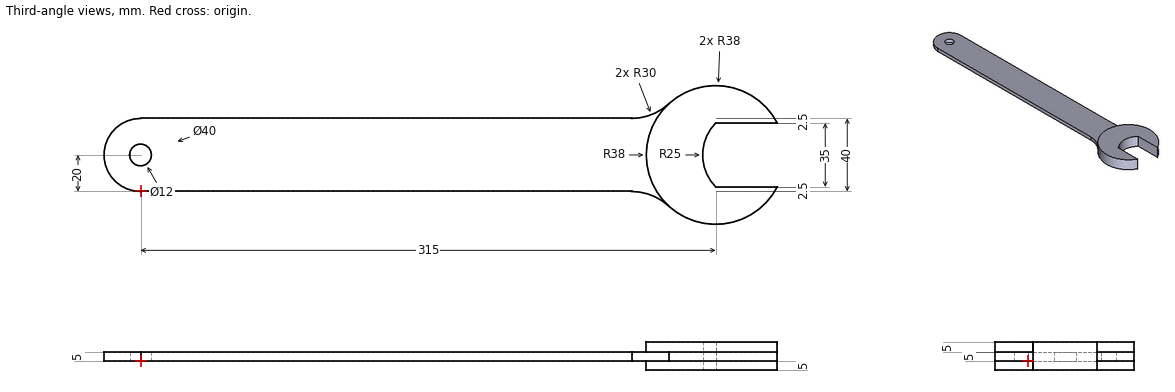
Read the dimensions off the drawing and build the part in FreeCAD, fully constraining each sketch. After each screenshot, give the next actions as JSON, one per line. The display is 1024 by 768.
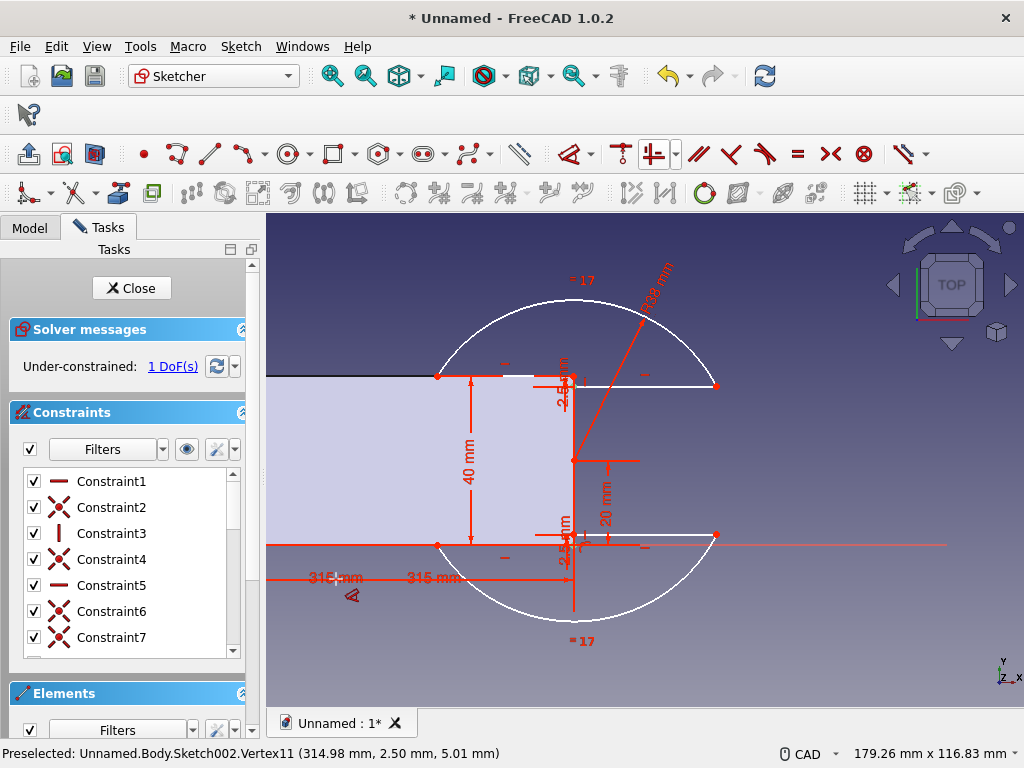
{"action": "left_click", "coordinate": [574, 461]}
{"action": "left_click", "coordinate": [532, 579]}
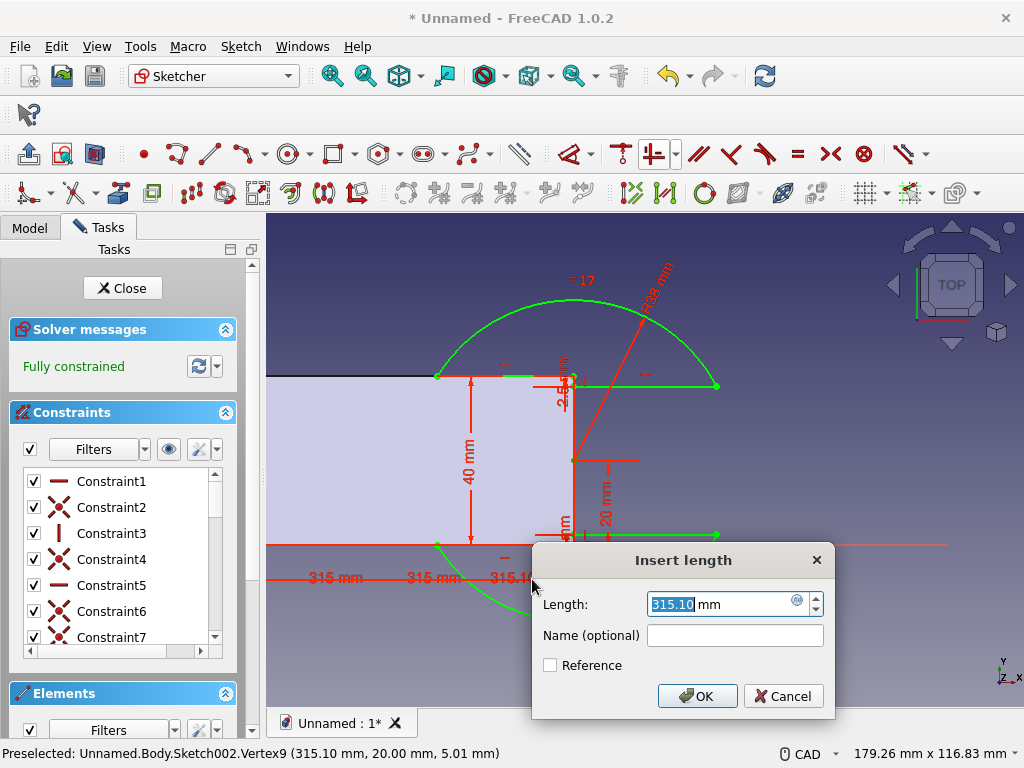
{"action": "type", "text": "315"}
{"action": "key", "text": "Return"}
{"action": "key", "text": "Escape"}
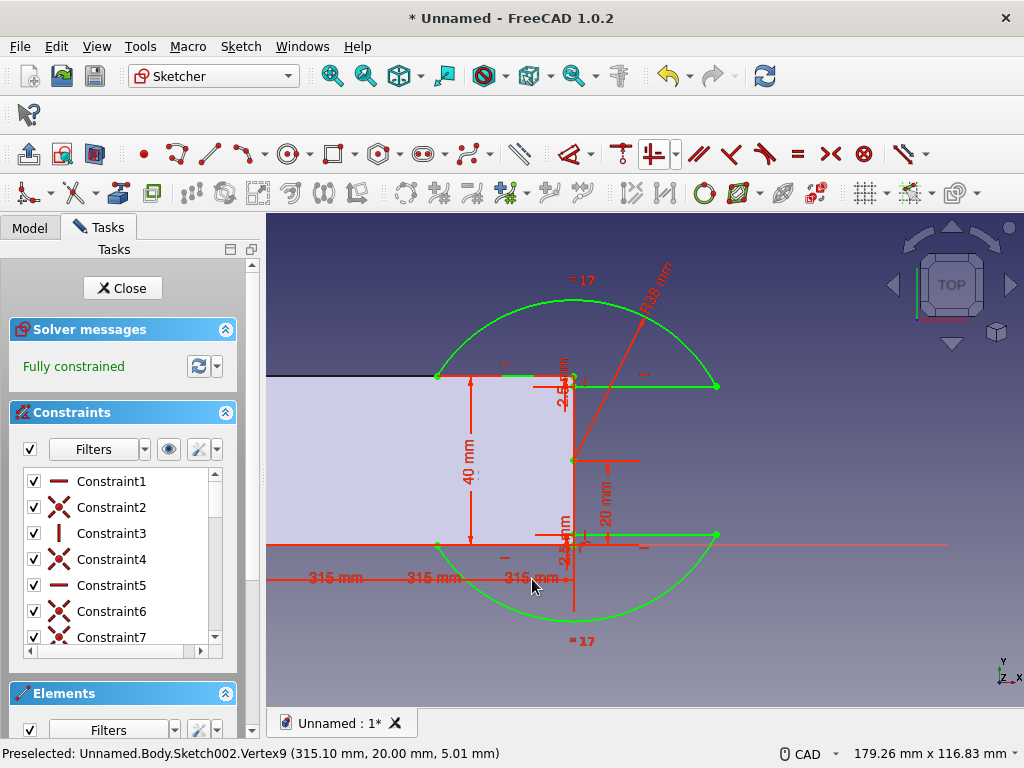
{"action": "left_click", "coordinate": [123, 288]}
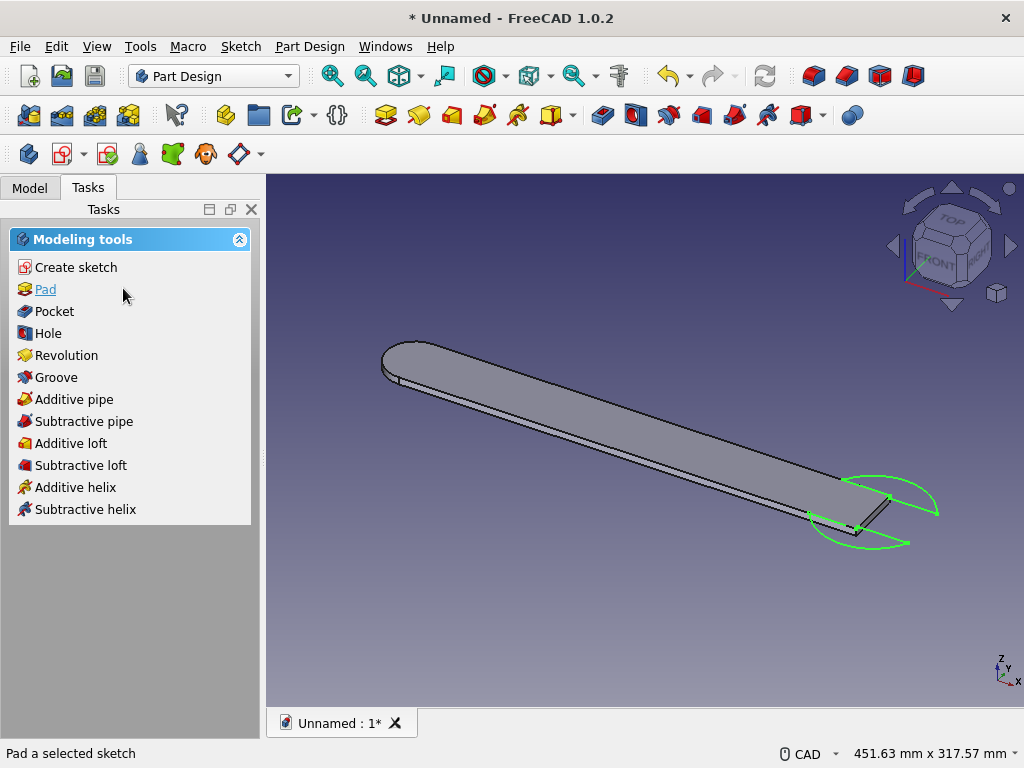
{"action": "left_click", "coordinate": [386, 116]}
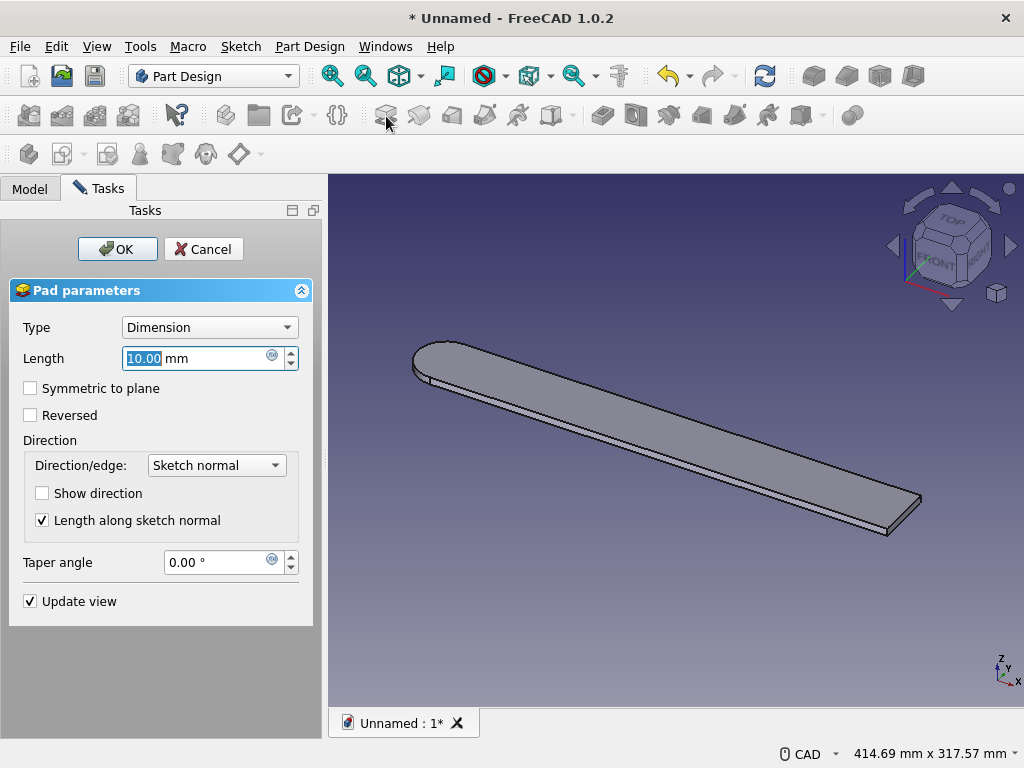
{"action": "type", "text": "5"}
{"action": "key", "text": "Tab"}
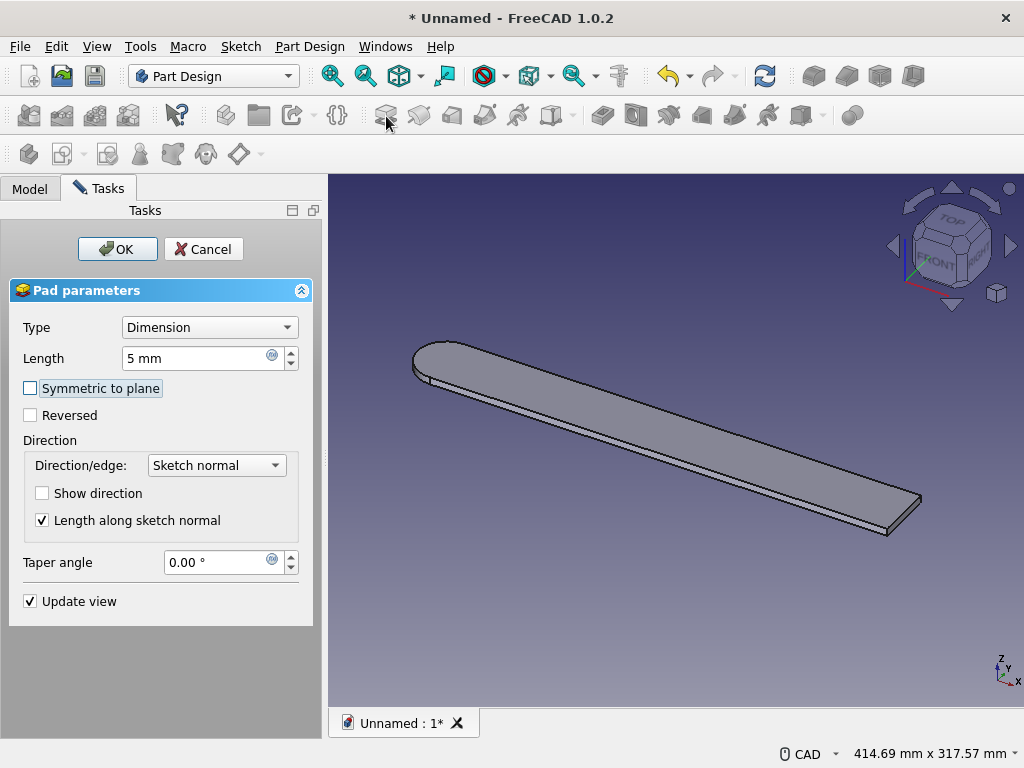
{"action": "left_click", "coordinate": [31, 415]}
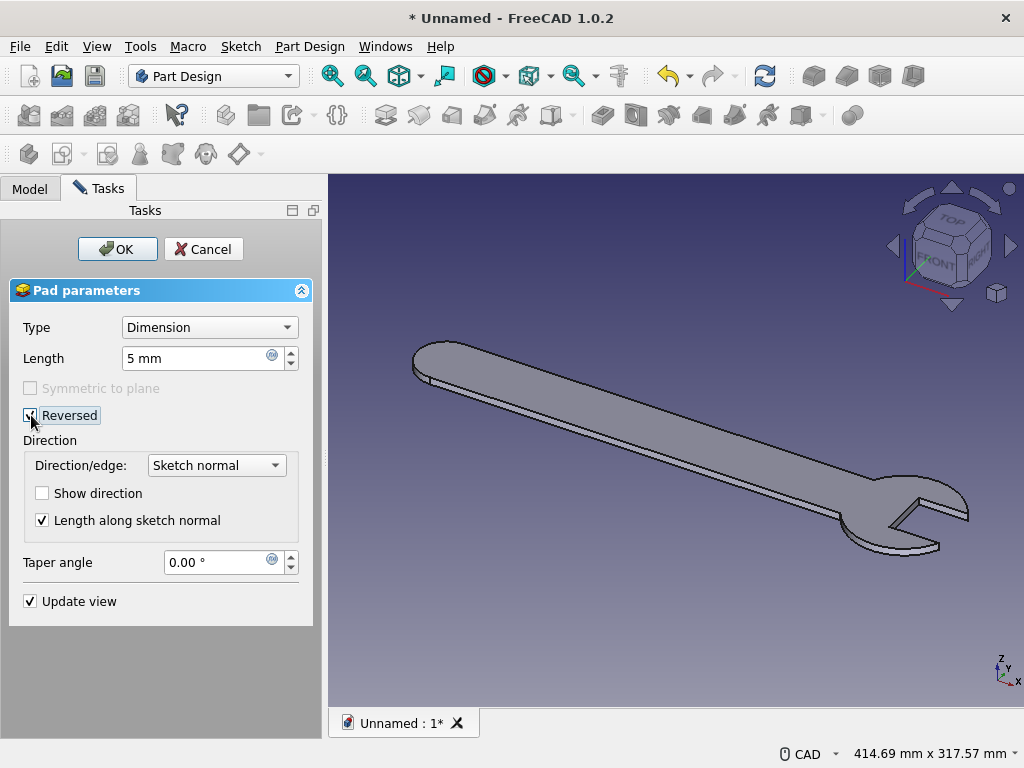
{"action": "left_click", "coordinate": [118, 249]}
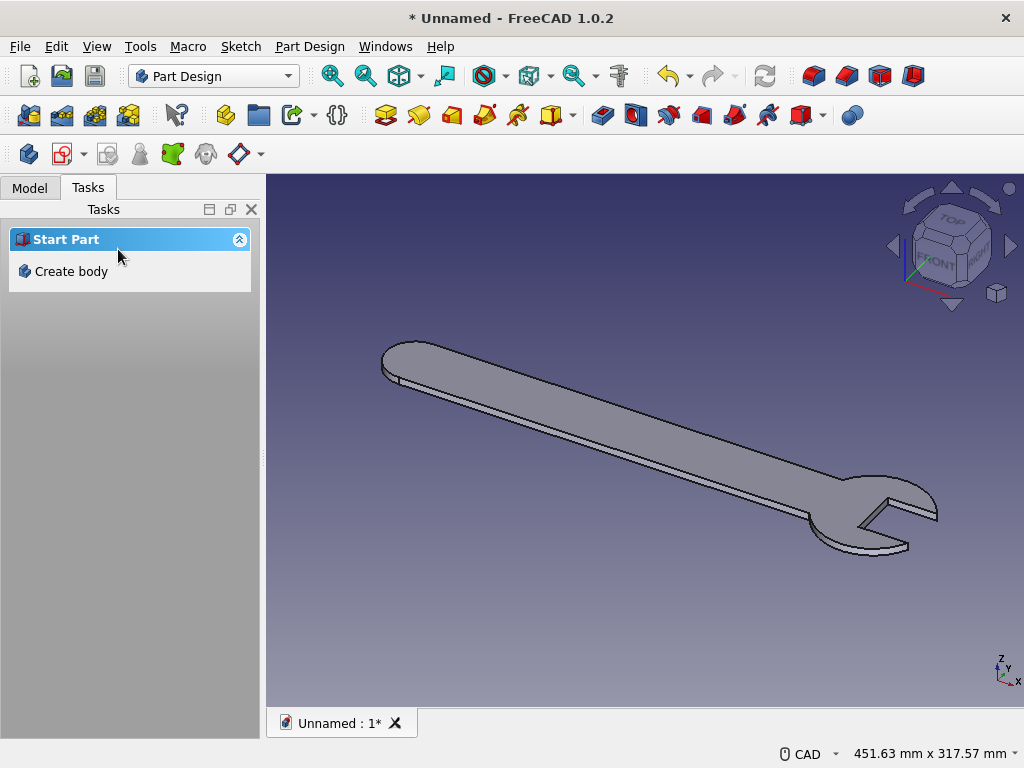
{"action": "left_click", "coordinate": [807, 489]}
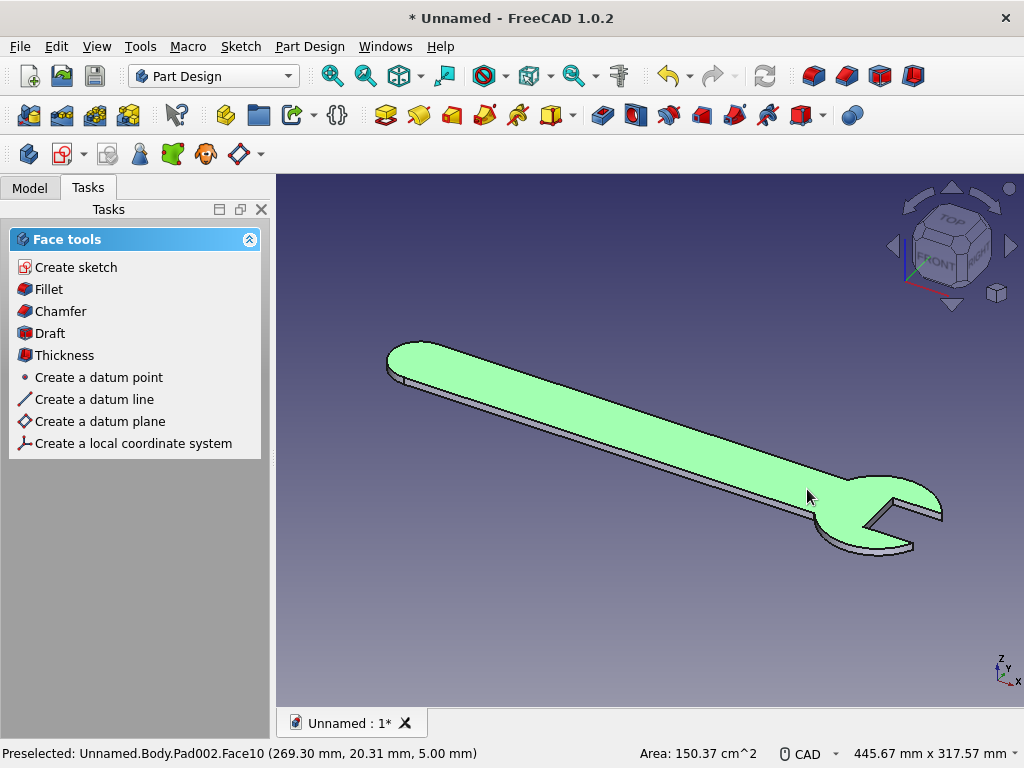
{"action": "left_click", "coordinate": [62, 154]}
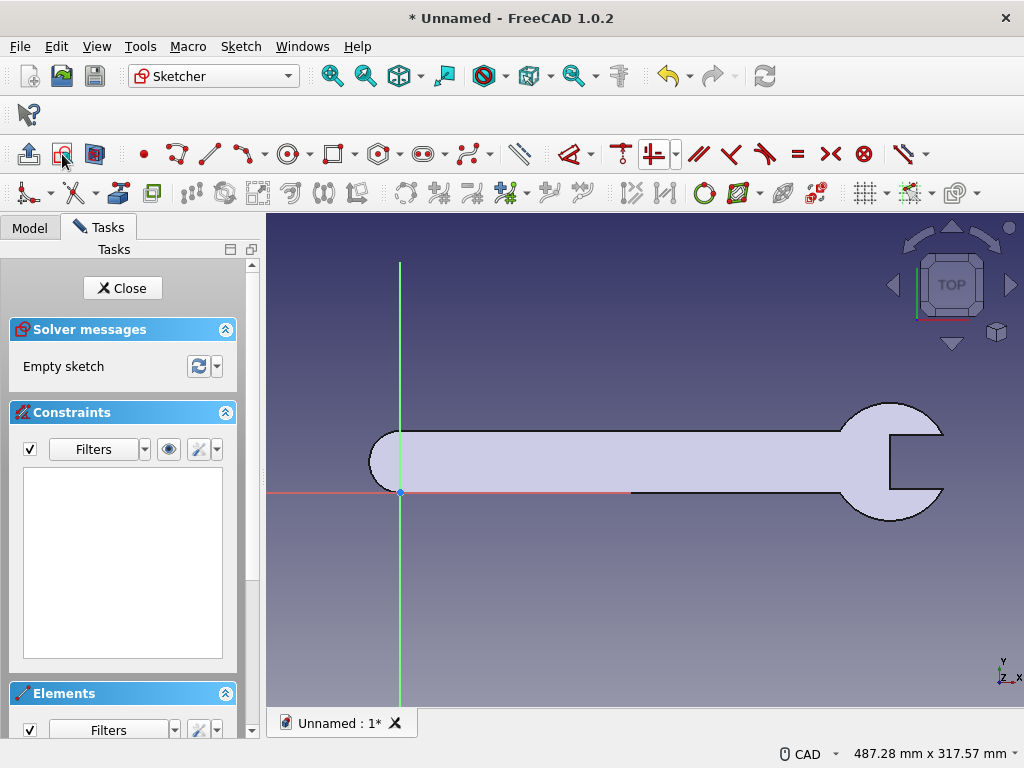
{"action": "scroll", "coordinate": [576, 460], "scroll_direction": "down", "scroll_amount": 5}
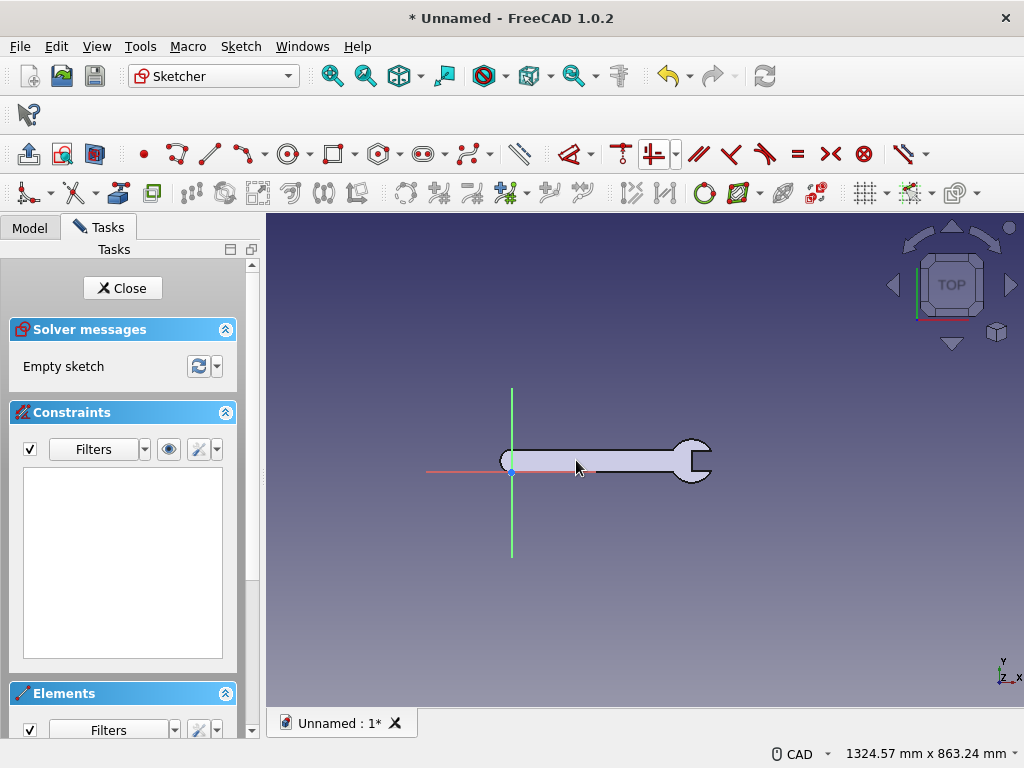
{"action": "scroll", "coordinate": [697, 461], "scroll_direction": "up", "scroll_amount": 14}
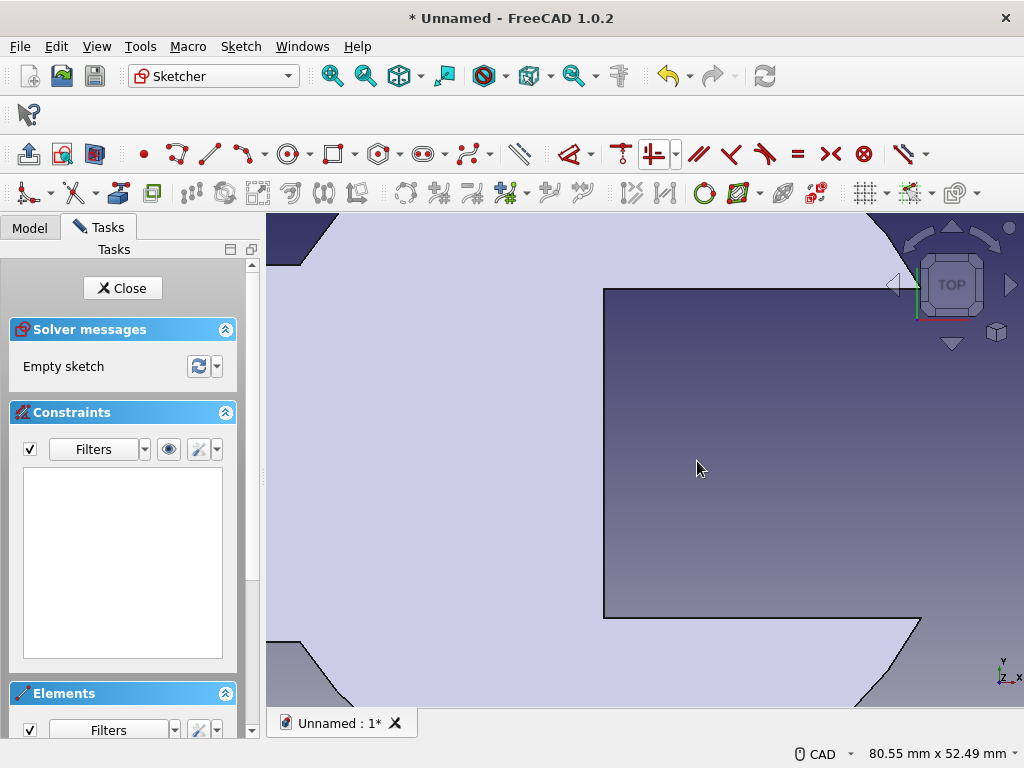
{"action": "left_click", "coordinate": [210, 154]}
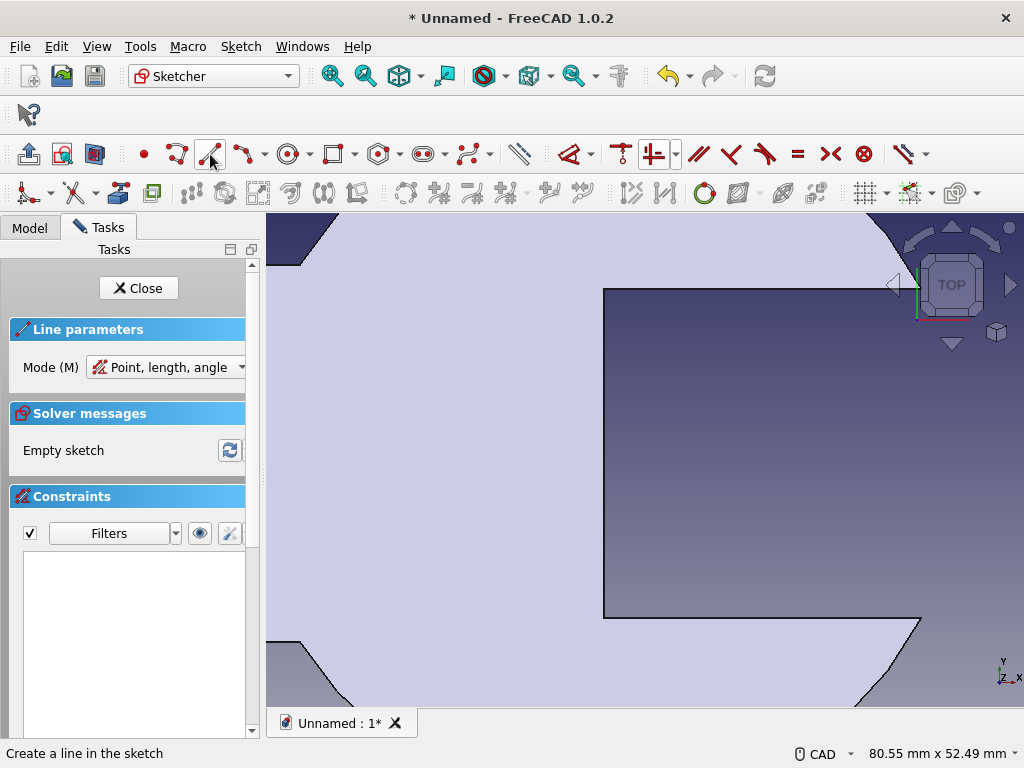
{"action": "left_click", "coordinate": [604, 618]}
{"action": "left_click", "coordinate": [604, 289]}